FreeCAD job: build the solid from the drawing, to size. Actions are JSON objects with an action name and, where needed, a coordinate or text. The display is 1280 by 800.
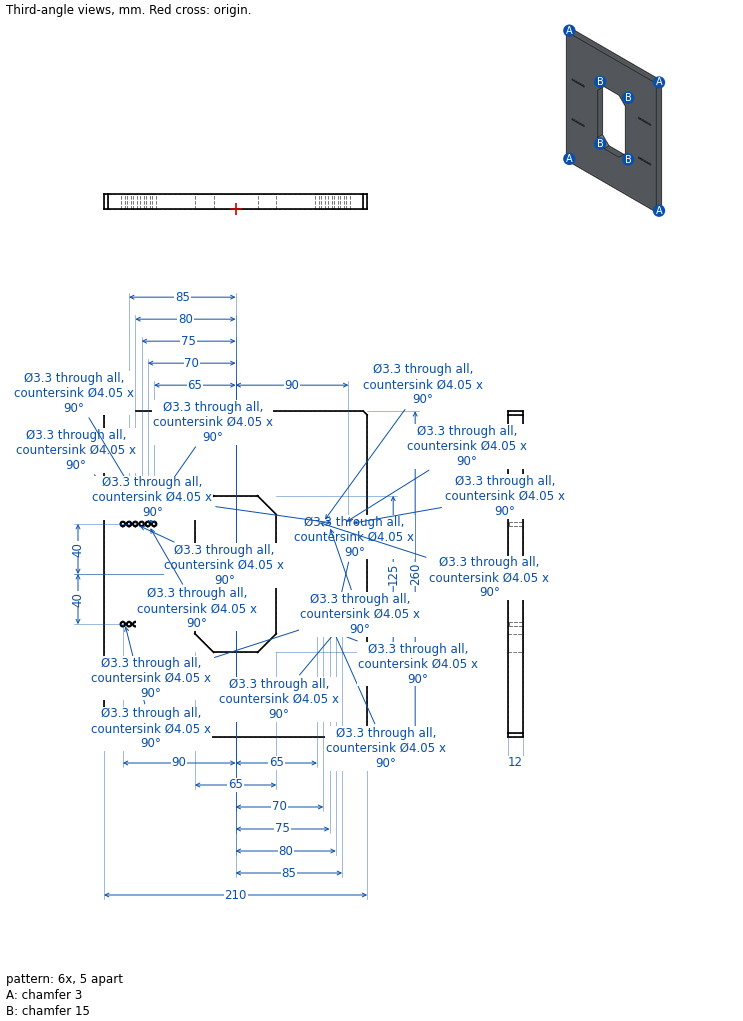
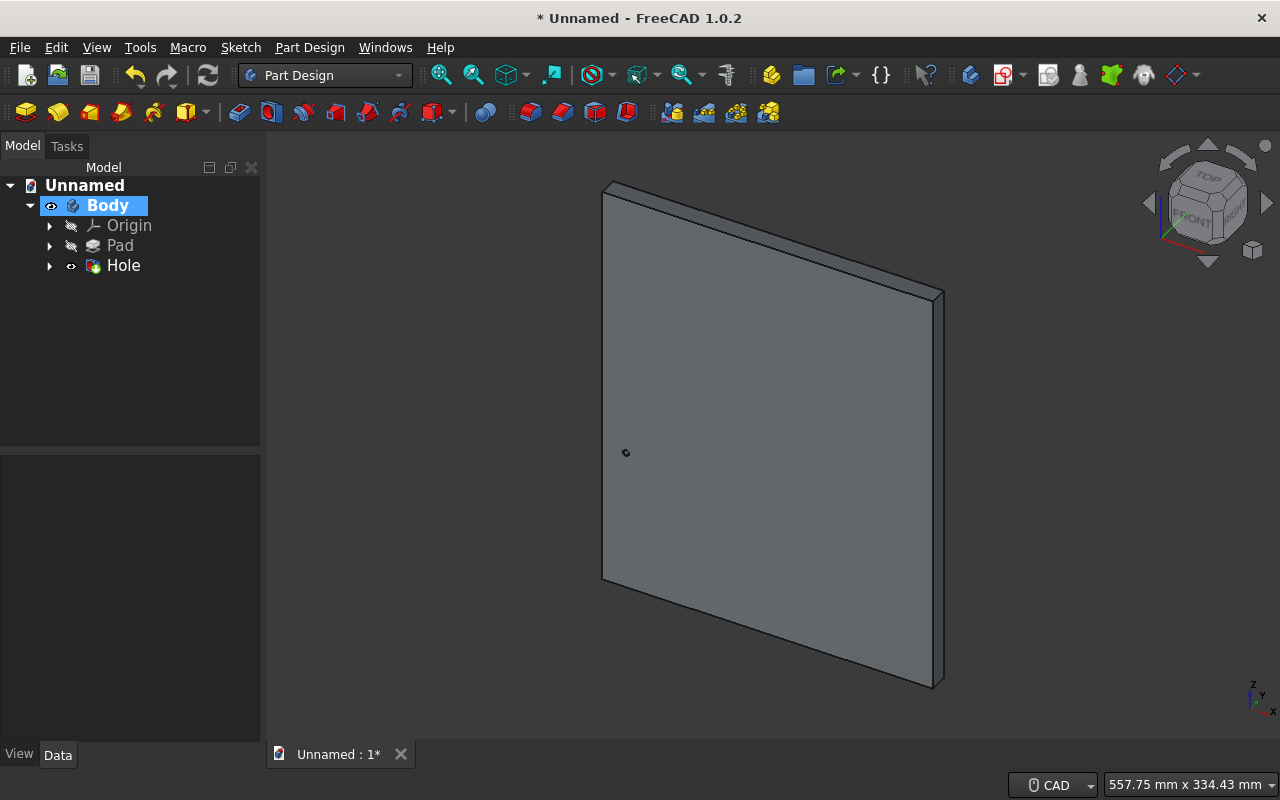
{"action": "left_click", "coordinate": [116, 266]}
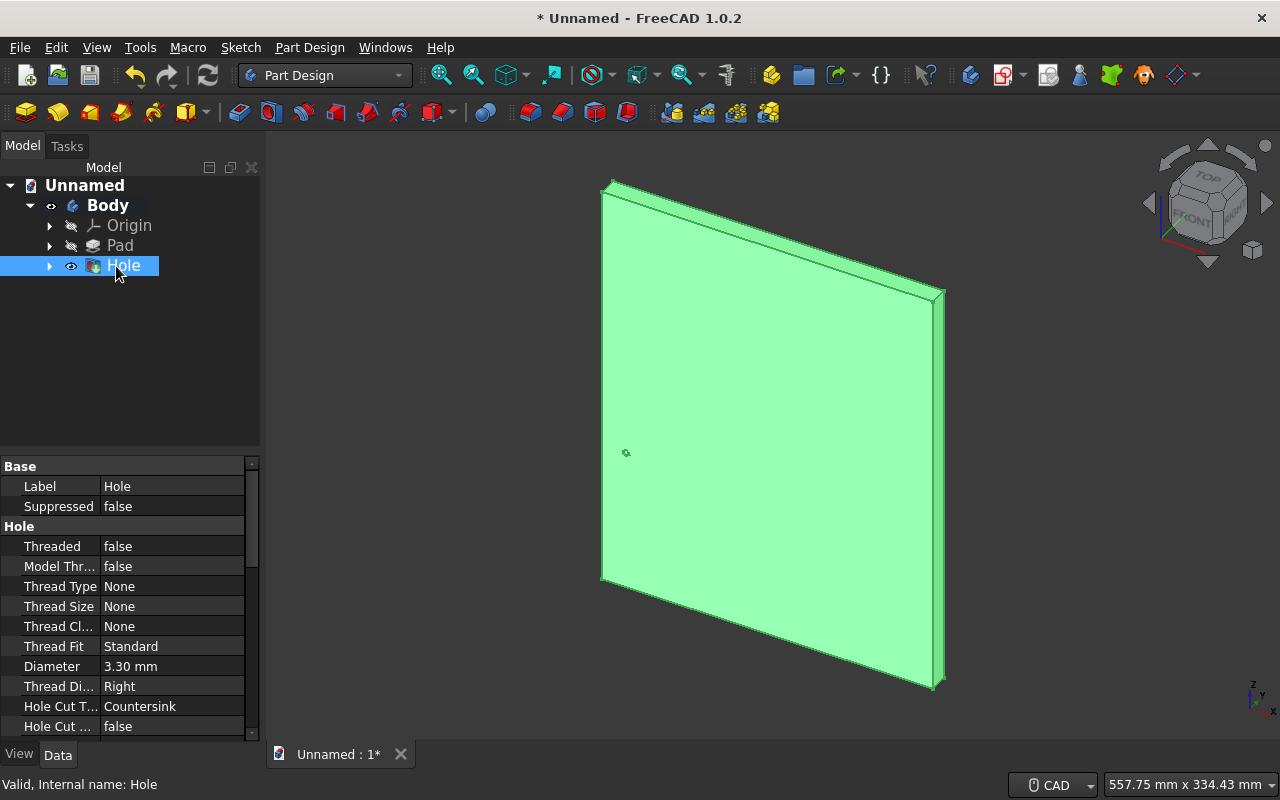
{"action": "left_click", "coordinate": [704, 112]}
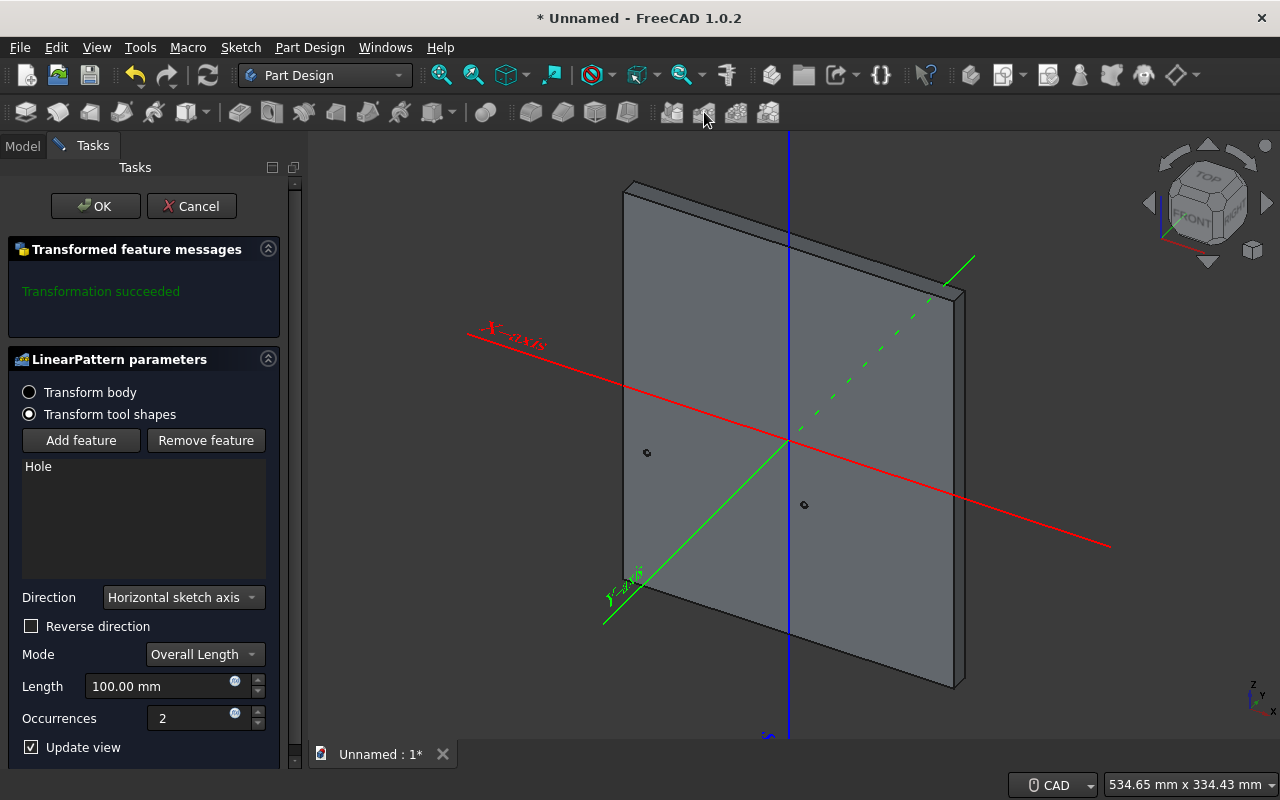
{"action": "left_click", "coordinate": [184, 598]}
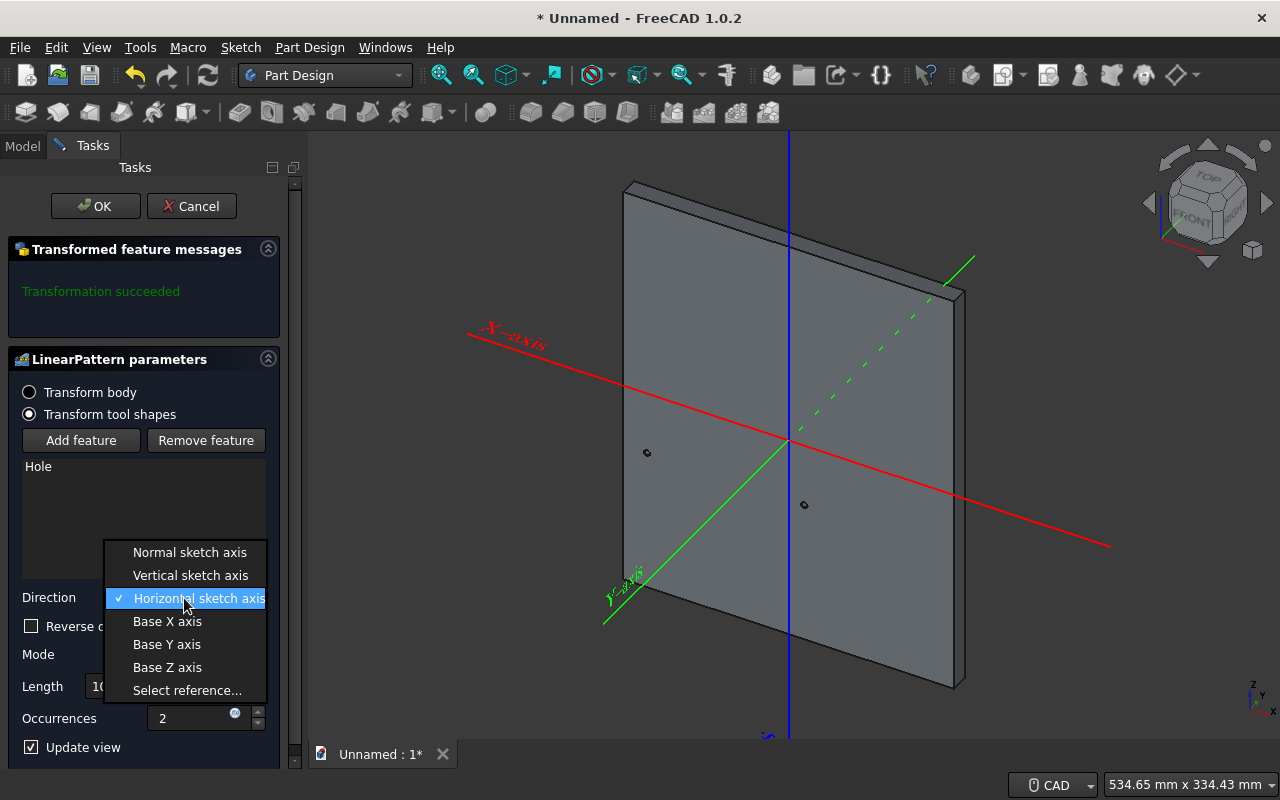
{"action": "left_click", "coordinate": [184, 622]}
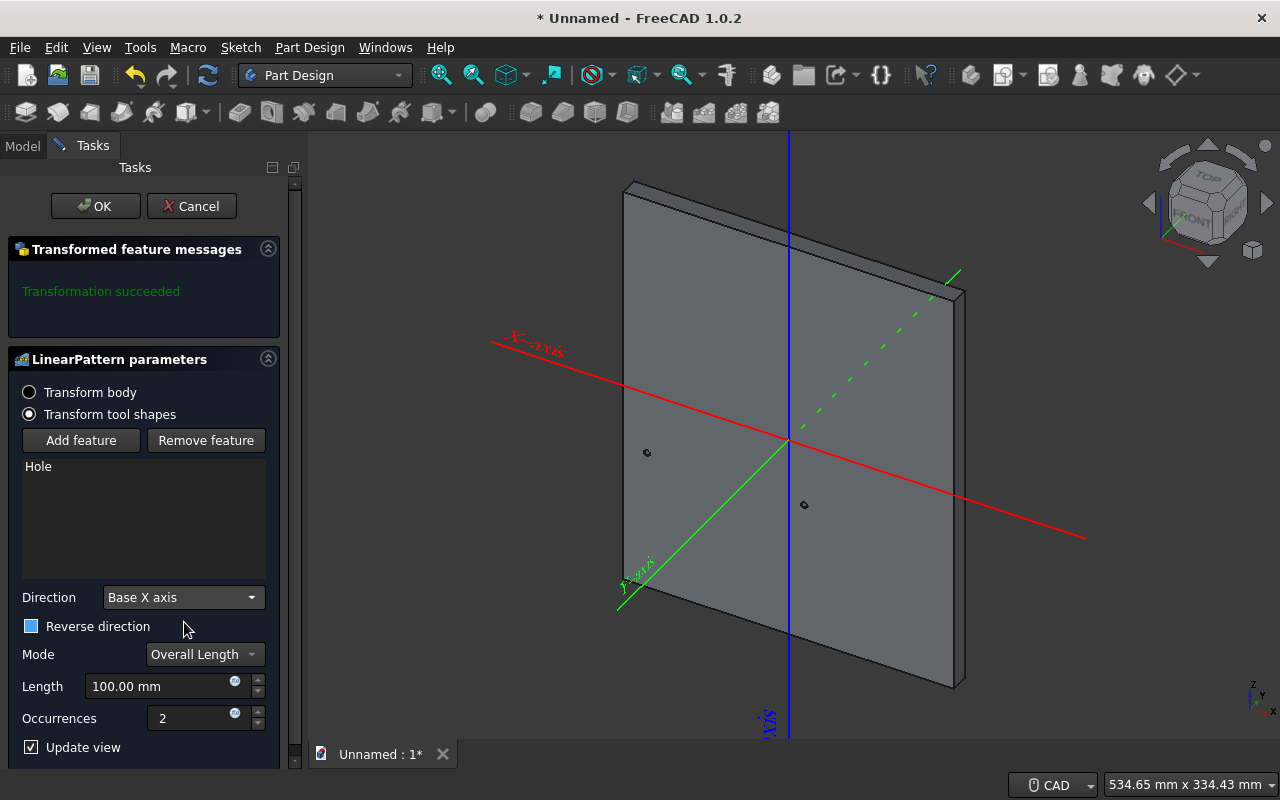
{"action": "left_click", "coordinate": [206, 654]}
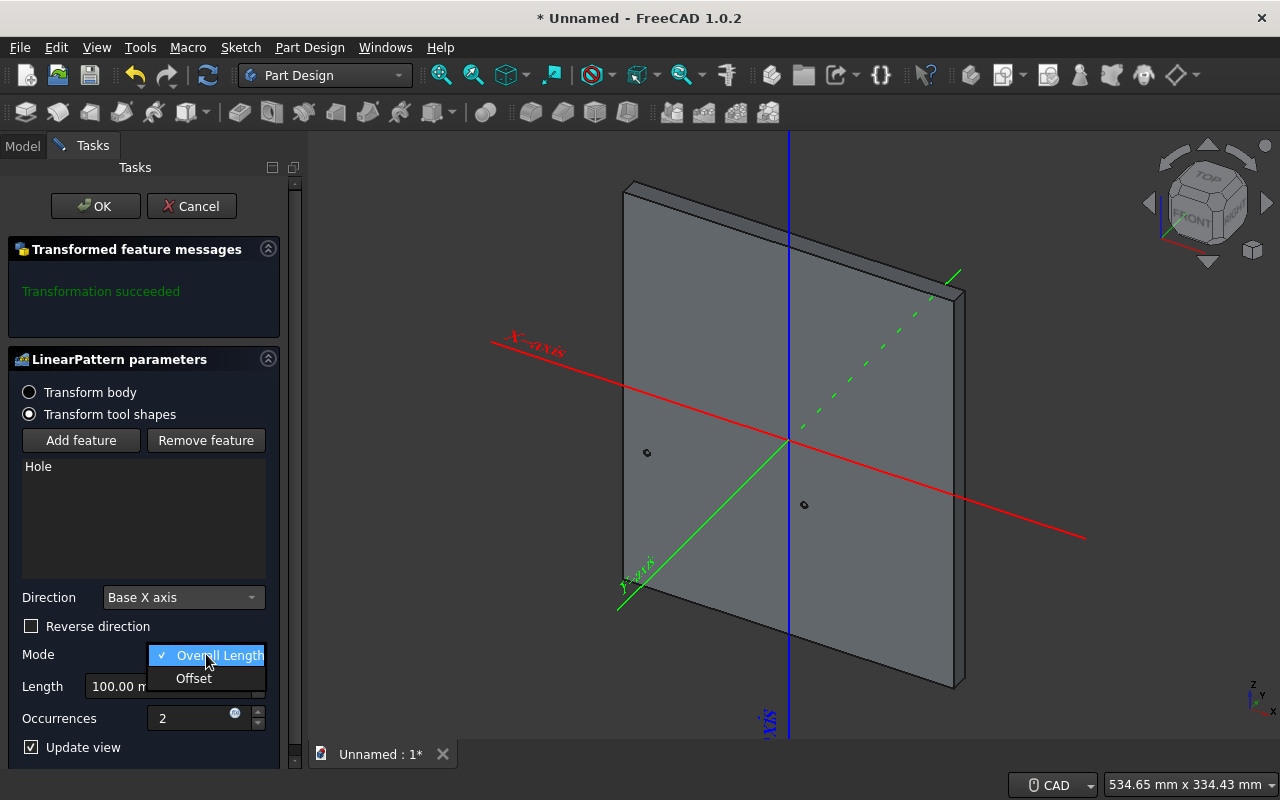
{"action": "left_click", "coordinate": [206, 678]}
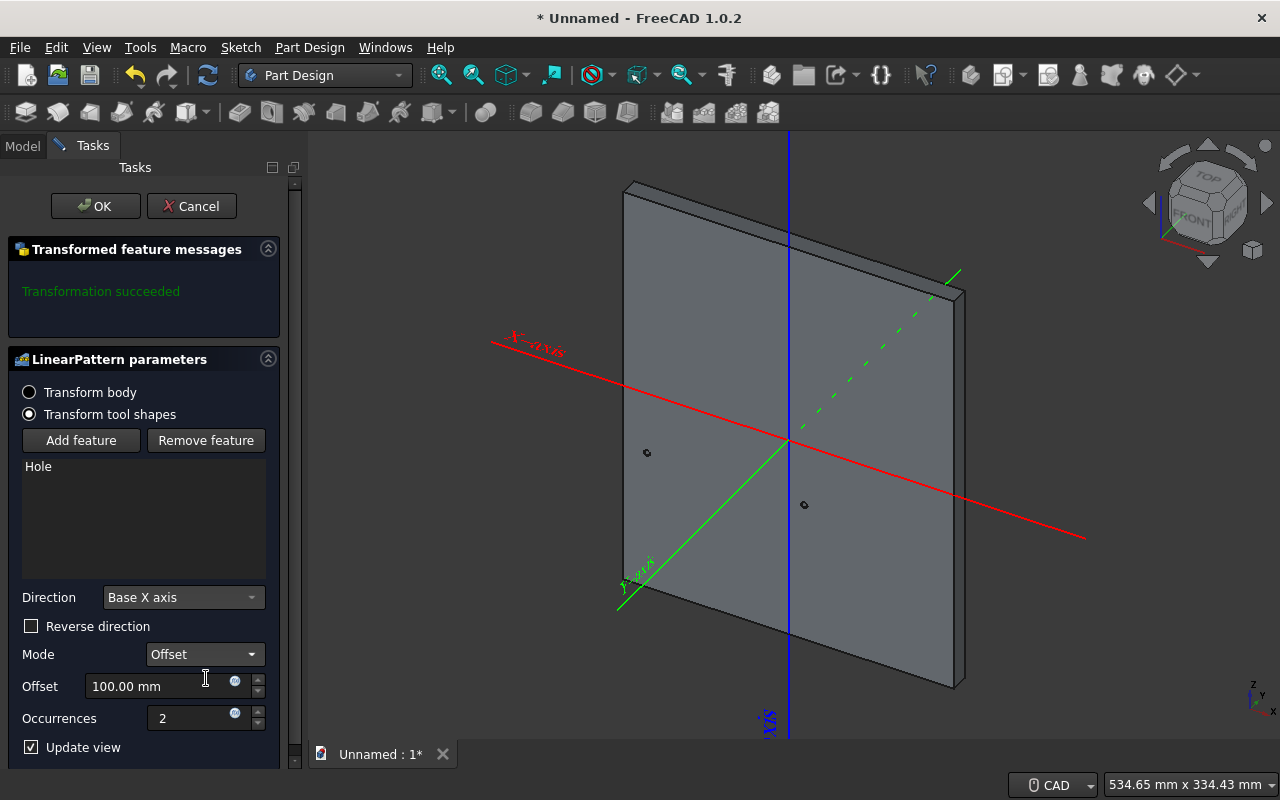
{"action": "triple_click", "coordinate": [168, 686]}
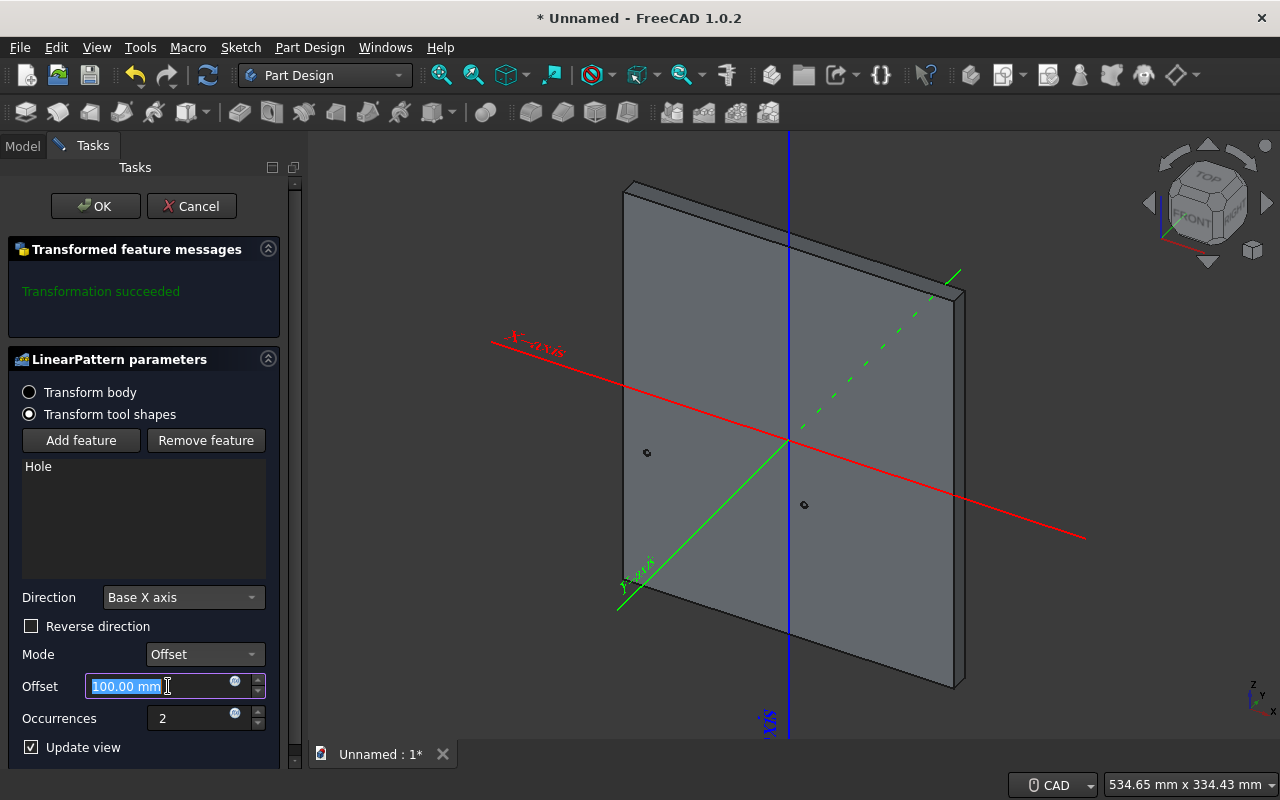
{"action": "type", "text": "5"}
{"action": "key", "text": "Tab"}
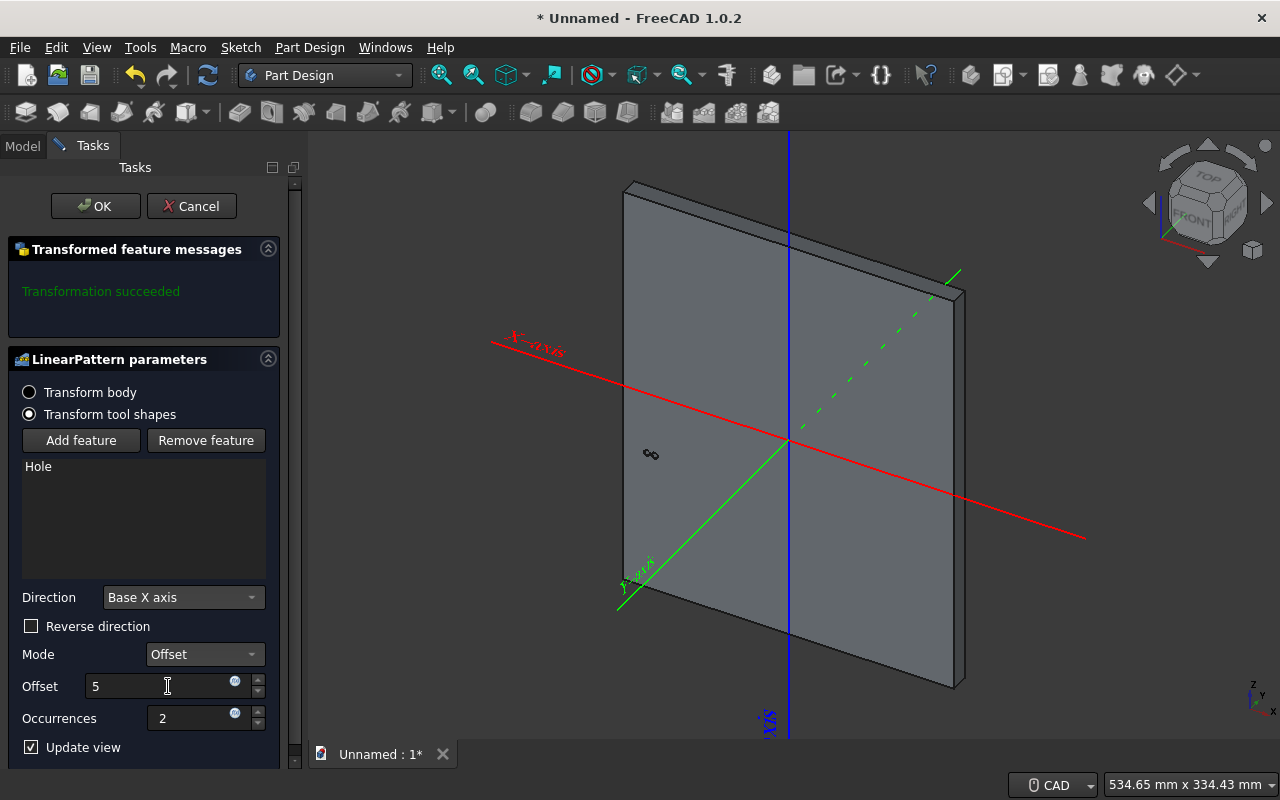
{"action": "triple_click", "coordinate": [198, 718]}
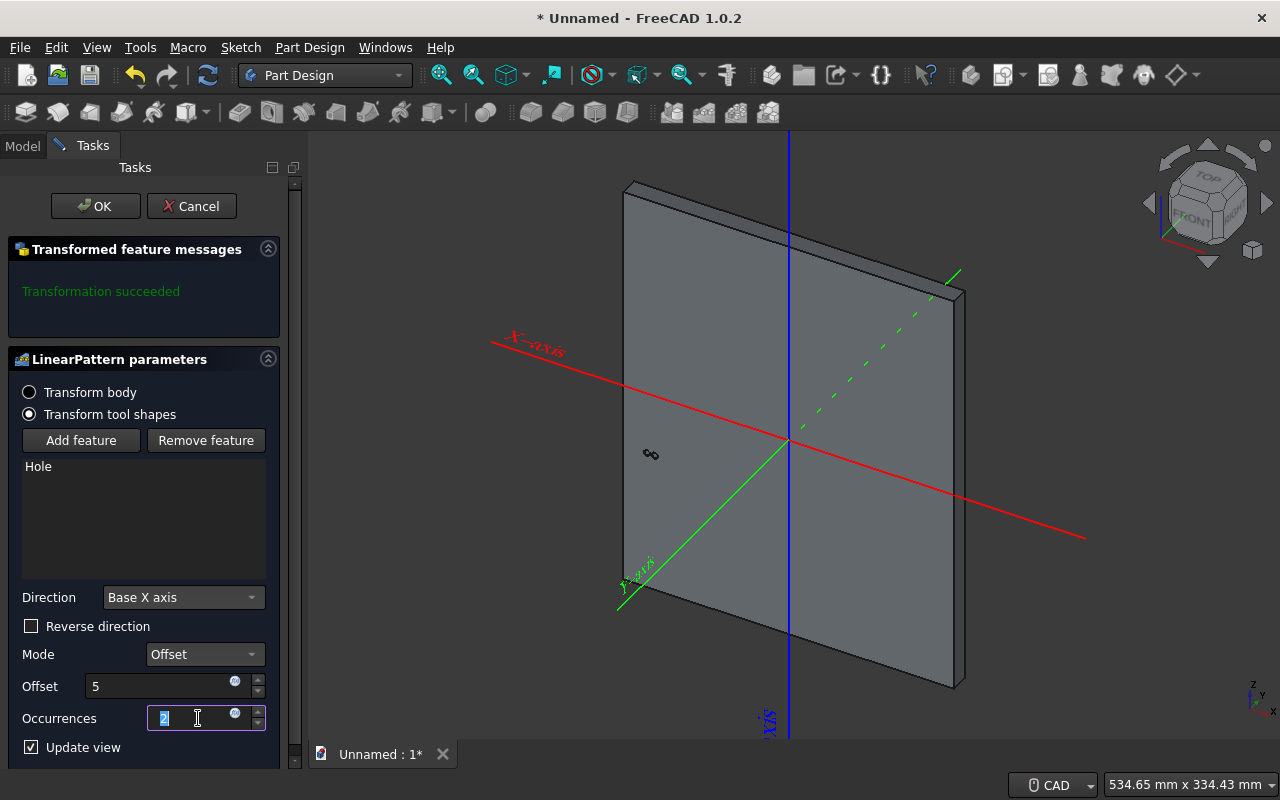
{"action": "type", "text": "6"}
{"action": "key", "text": "Tab"}